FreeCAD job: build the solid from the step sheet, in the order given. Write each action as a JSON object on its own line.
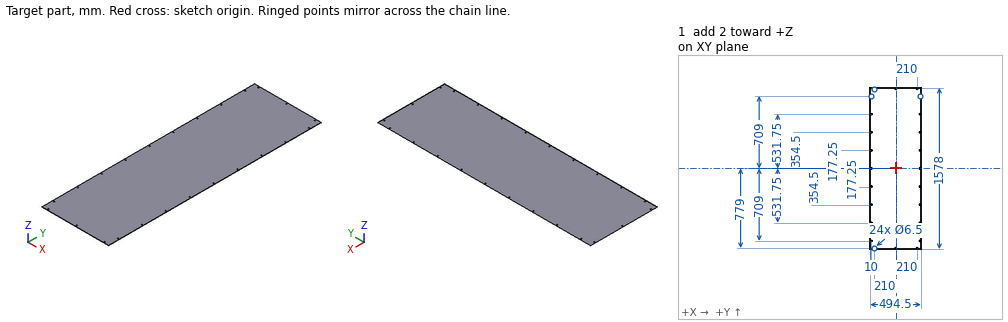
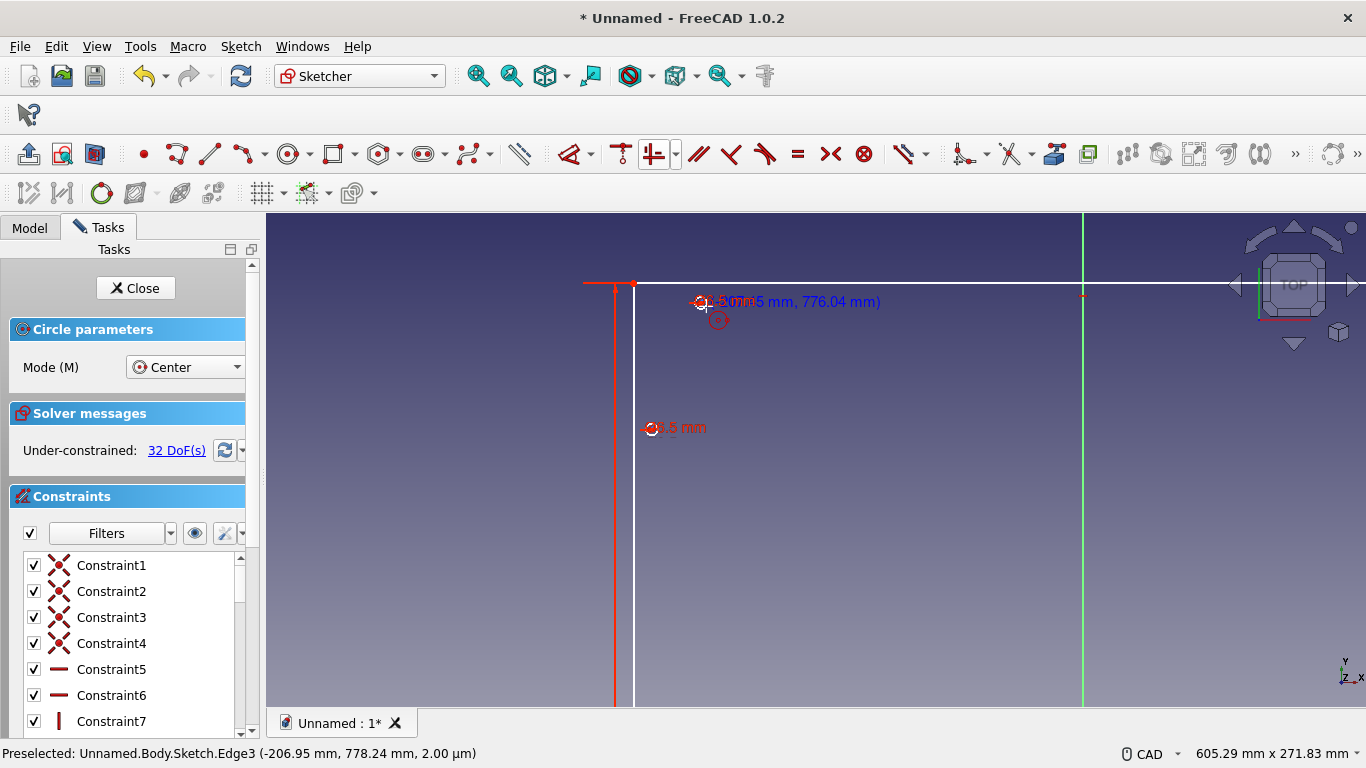
{"action": "scroll", "coordinate": [706, 303], "scroll_direction": "down", "scroll_amount": 11}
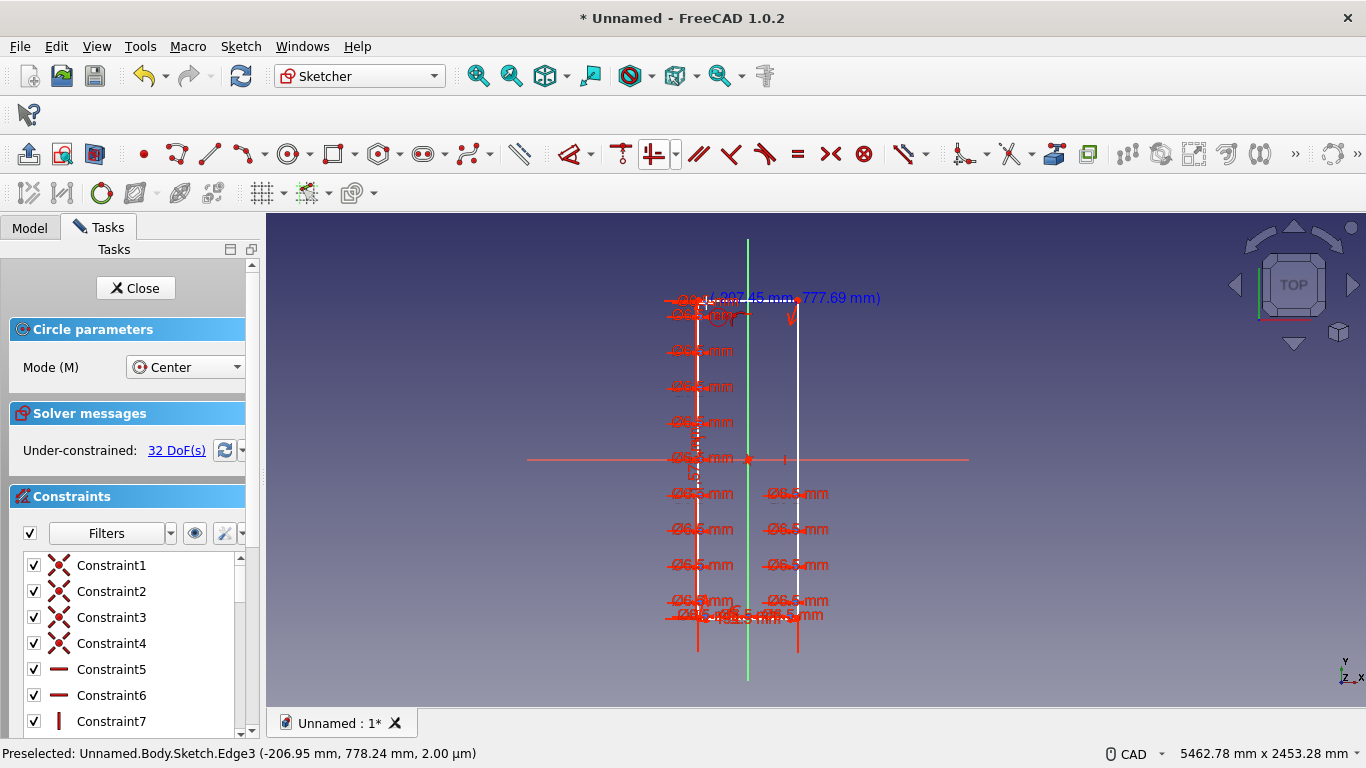
{"action": "scroll", "coordinate": [796, 460], "scroll_direction": "up", "scroll_amount": 18}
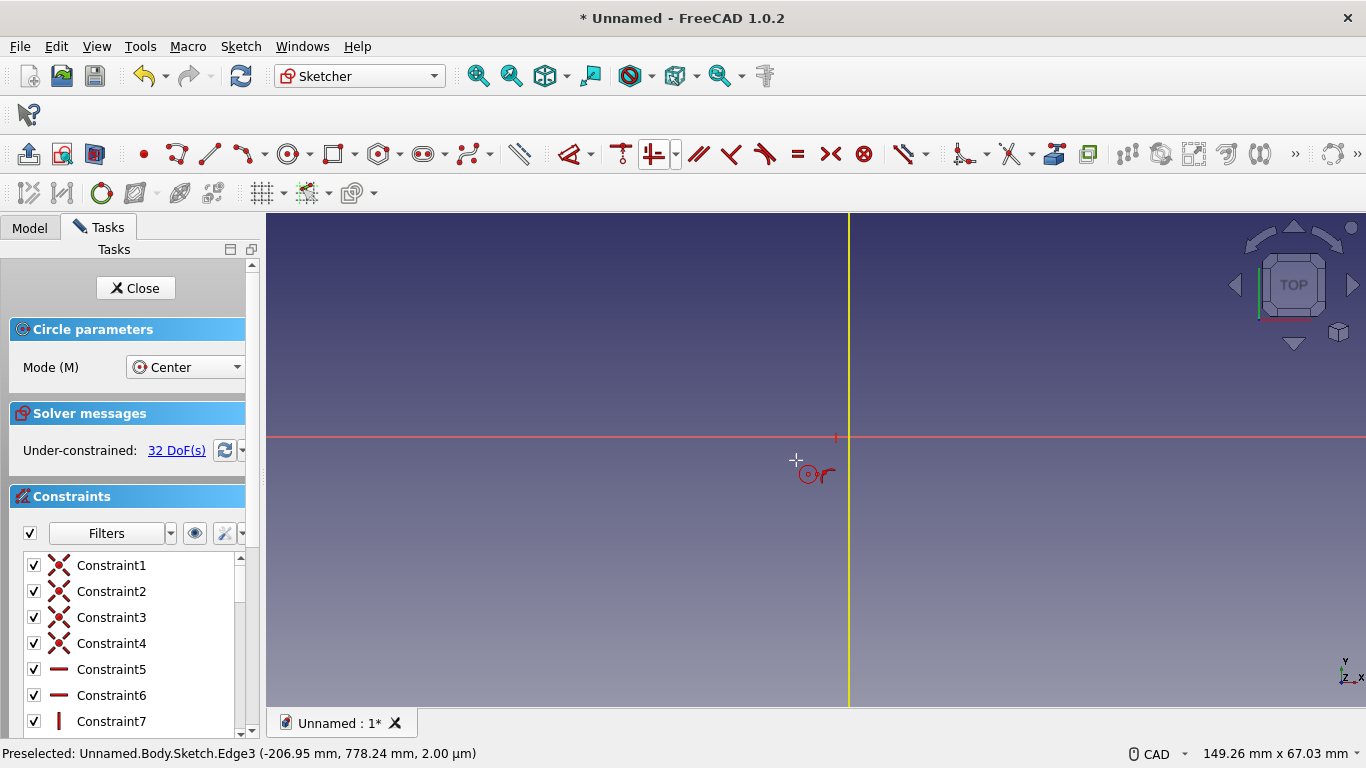
{"action": "scroll", "coordinate": [796, 461], "scroll_direction": "down", "scroll_amount": 18}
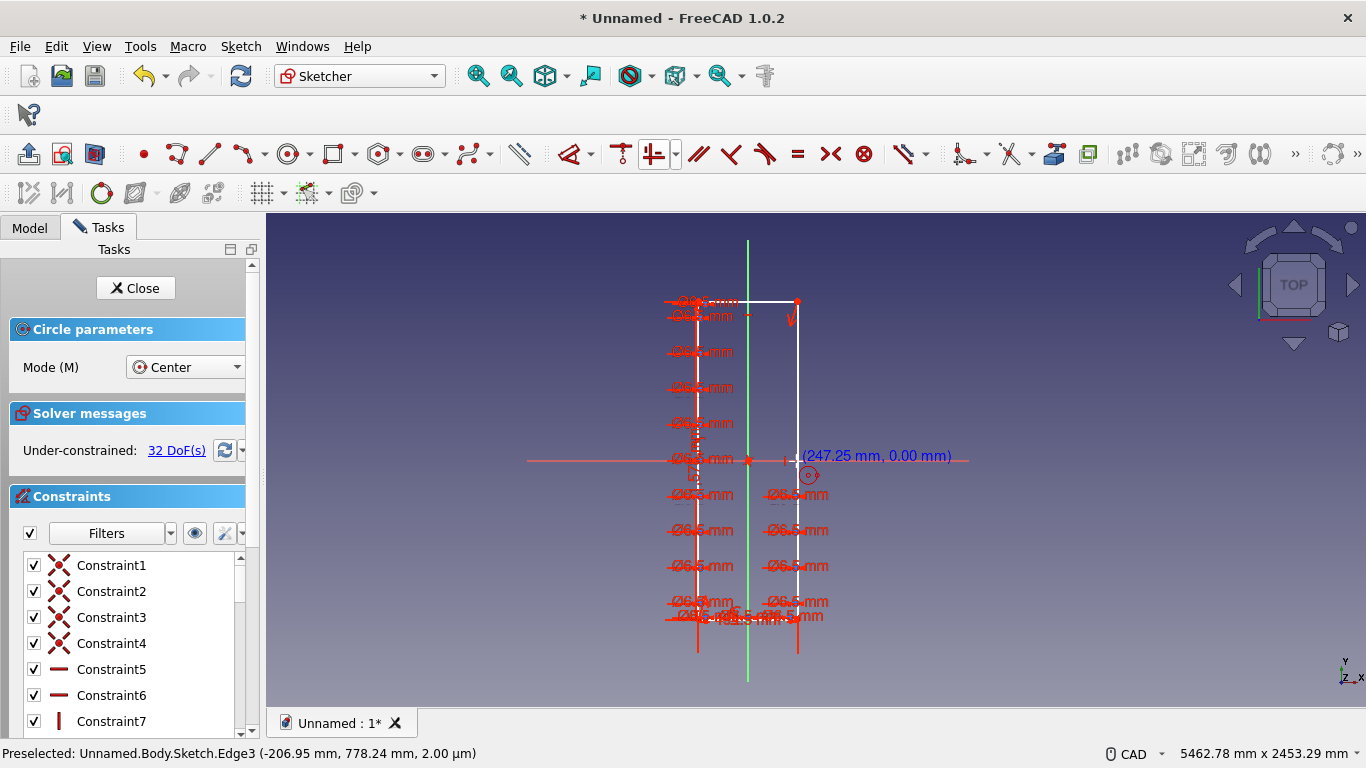
{"action": "scroll", "coordinate": [796, 461], "scroll_direction": "up", "scroll_amount": 11}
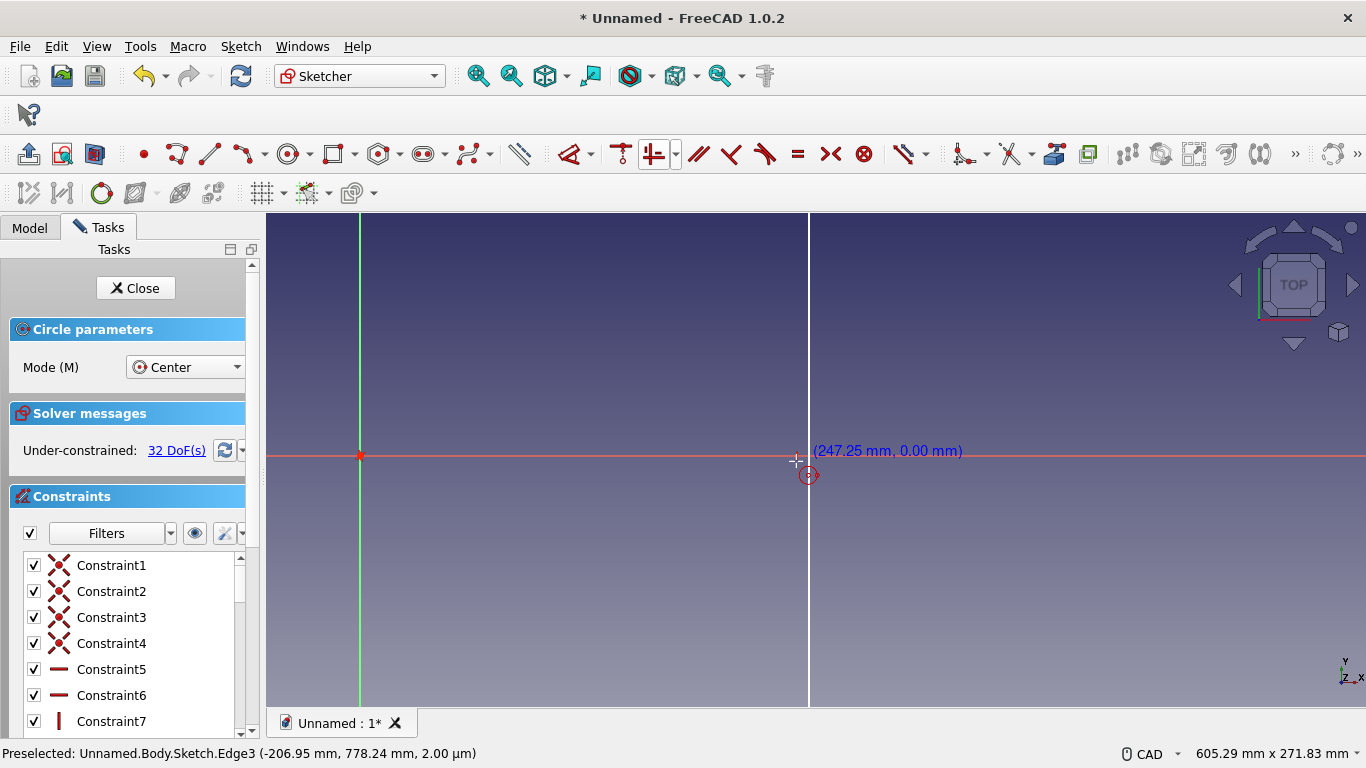
{"action": "left_click", "coordinate": [791, 456]}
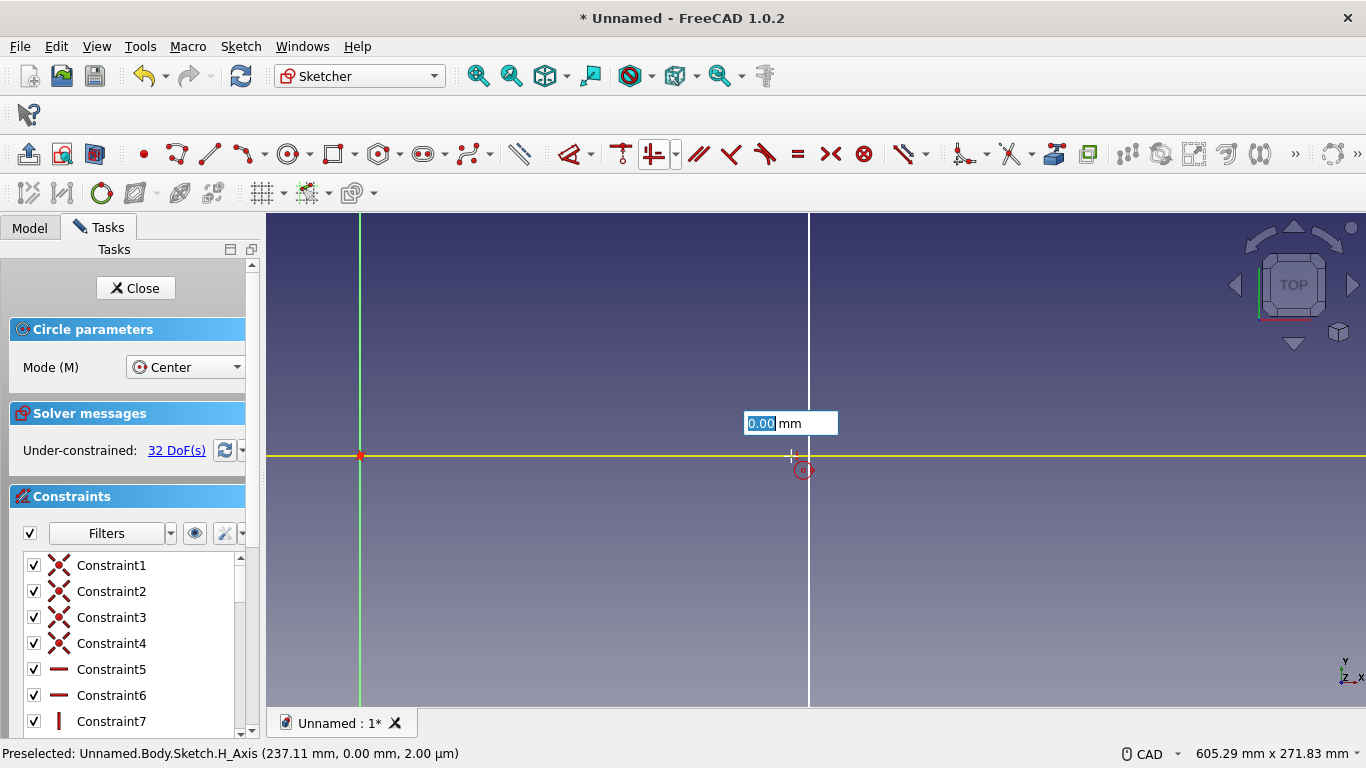
{"action": "scroll", "coordinate": [789, 461], "scroll_direction": "up", "scroll_amount": 6}
{"action": "mouse_move", "coordinate": [789, 460]}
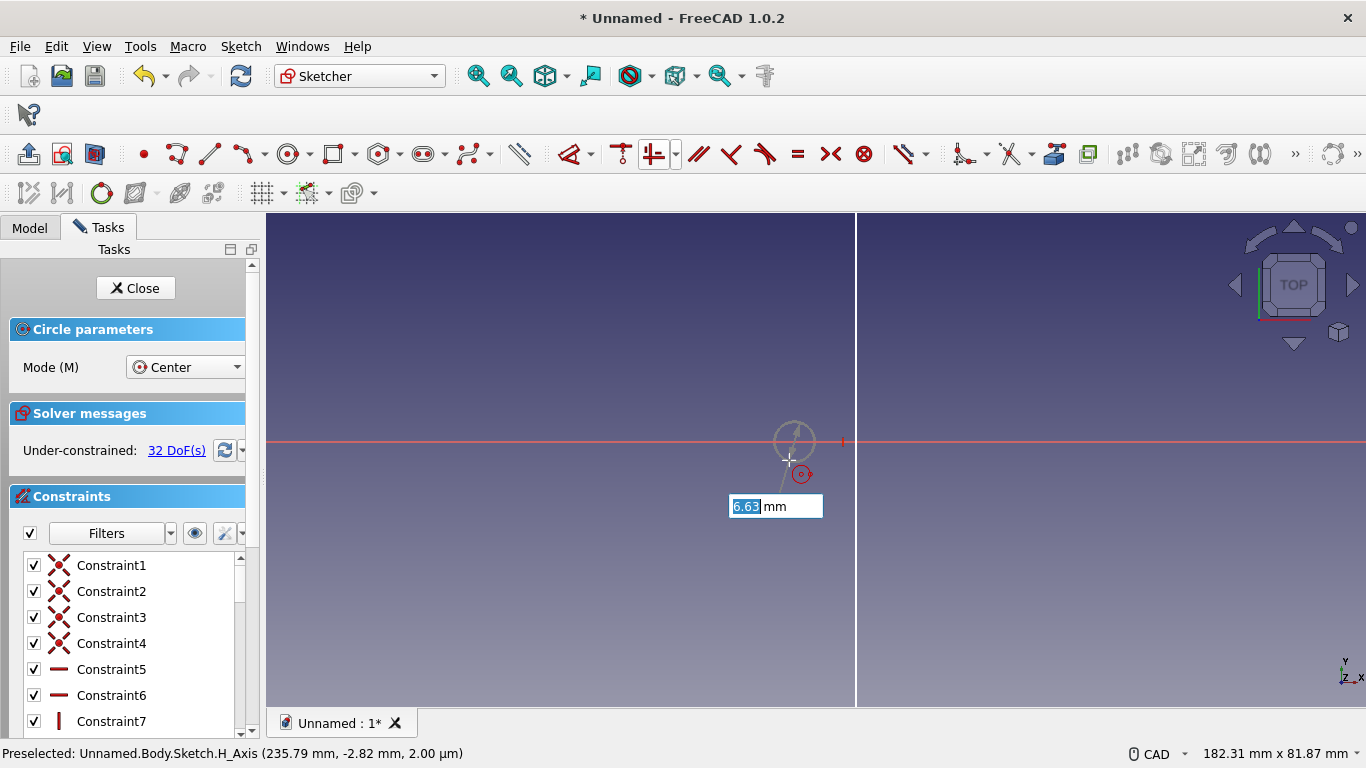
{"action": "type", "text": "6.5"}
{"action": "key", "text": "Return"}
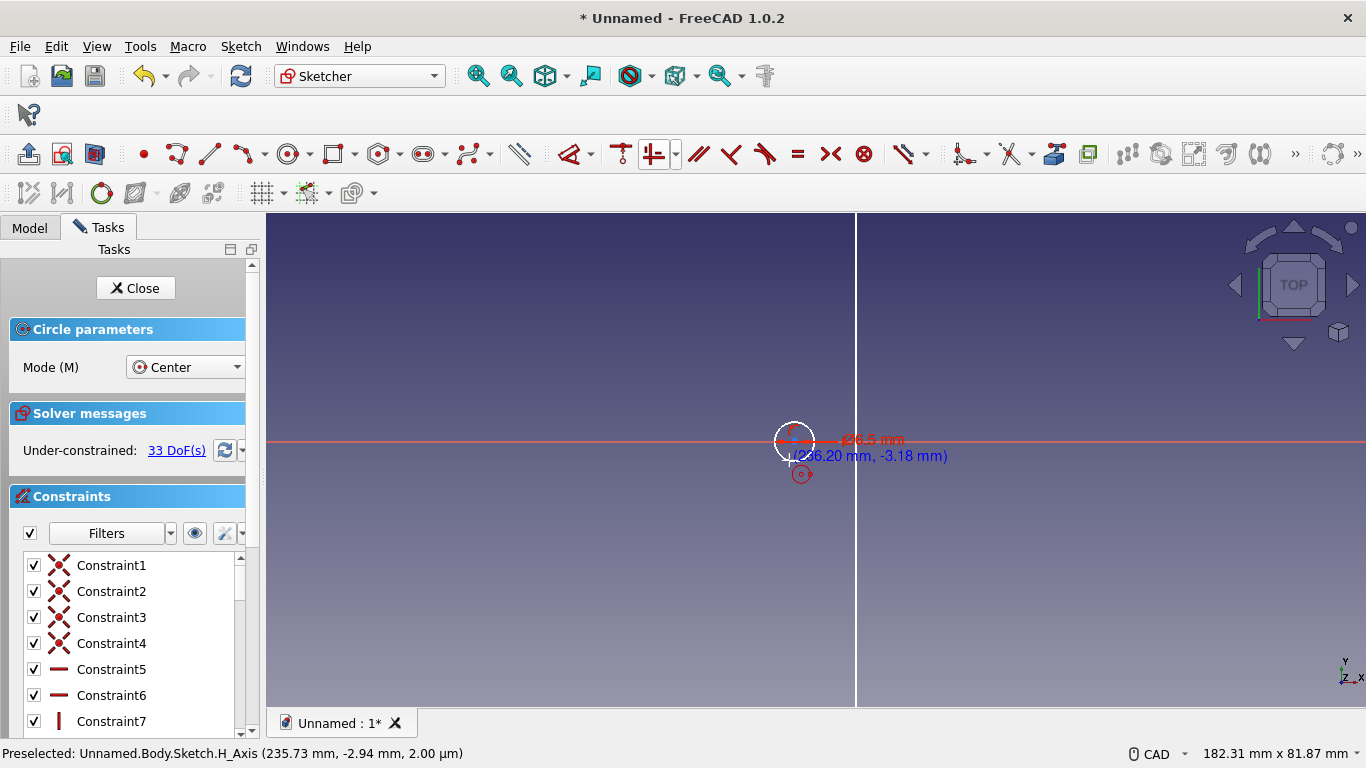
{"action": "scroll", "coordinate": [795, 461], "scroll_direction": "down", "scroll_amount": 17}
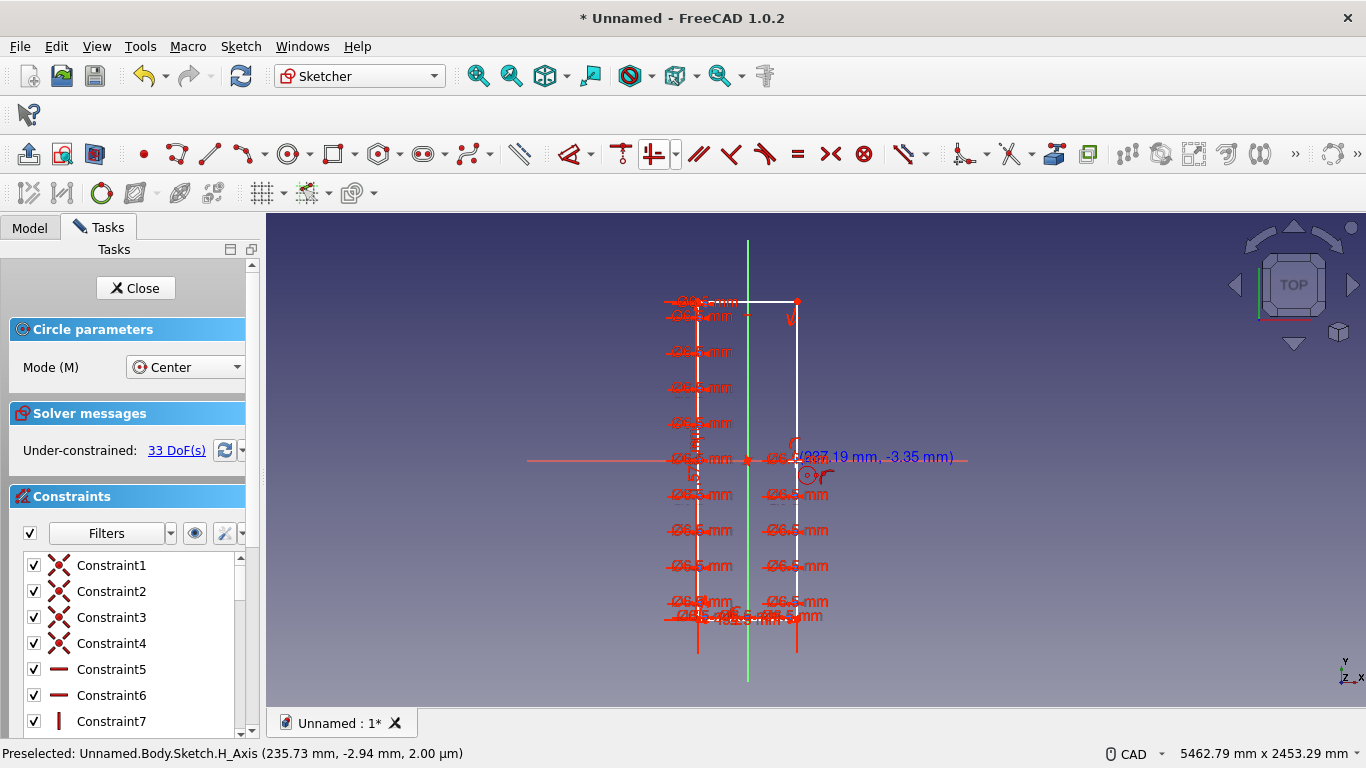
{"action": "scroll", "coordinate": [795, 425], "scroll_direction": "up", "scroll_amount": 18}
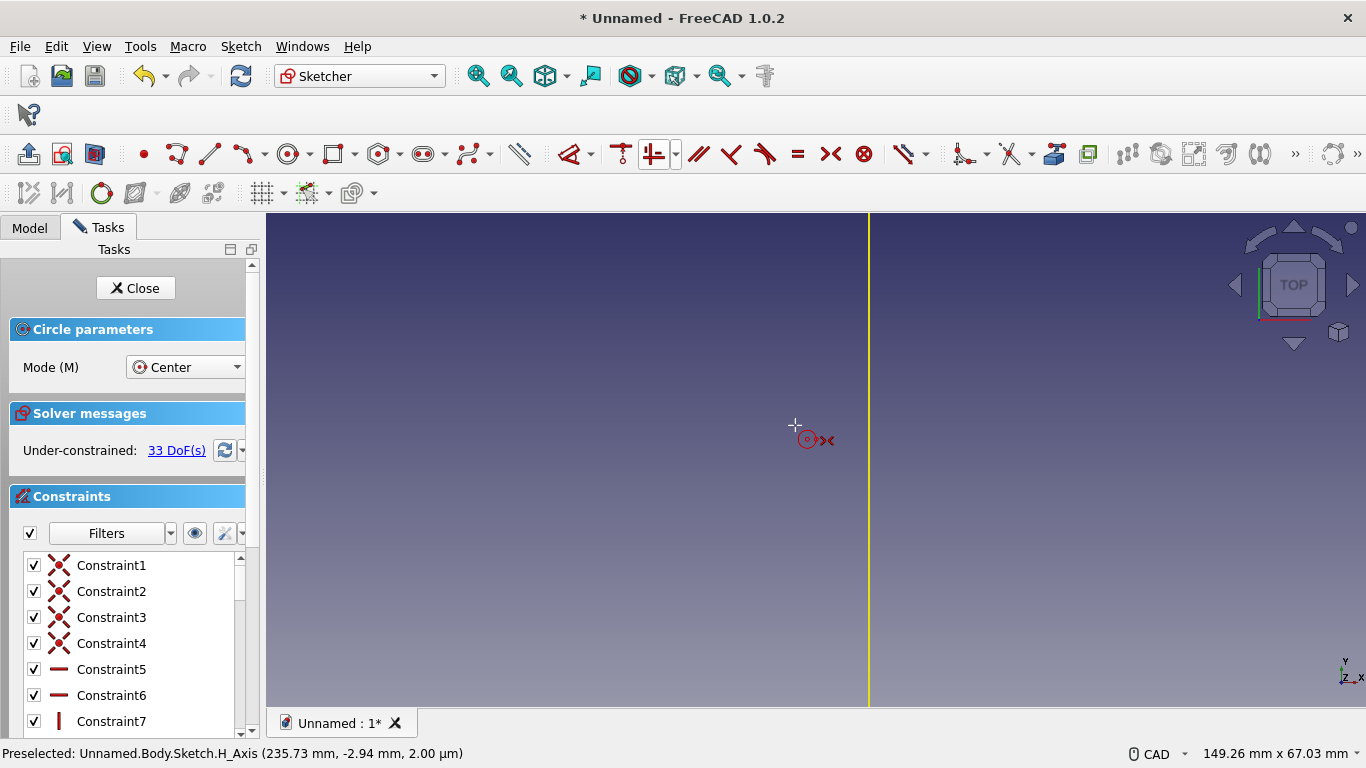
{"action": "scroll", "coordinate": [795, 425], "scroll_direction": "down", "scroll_amount": 18}